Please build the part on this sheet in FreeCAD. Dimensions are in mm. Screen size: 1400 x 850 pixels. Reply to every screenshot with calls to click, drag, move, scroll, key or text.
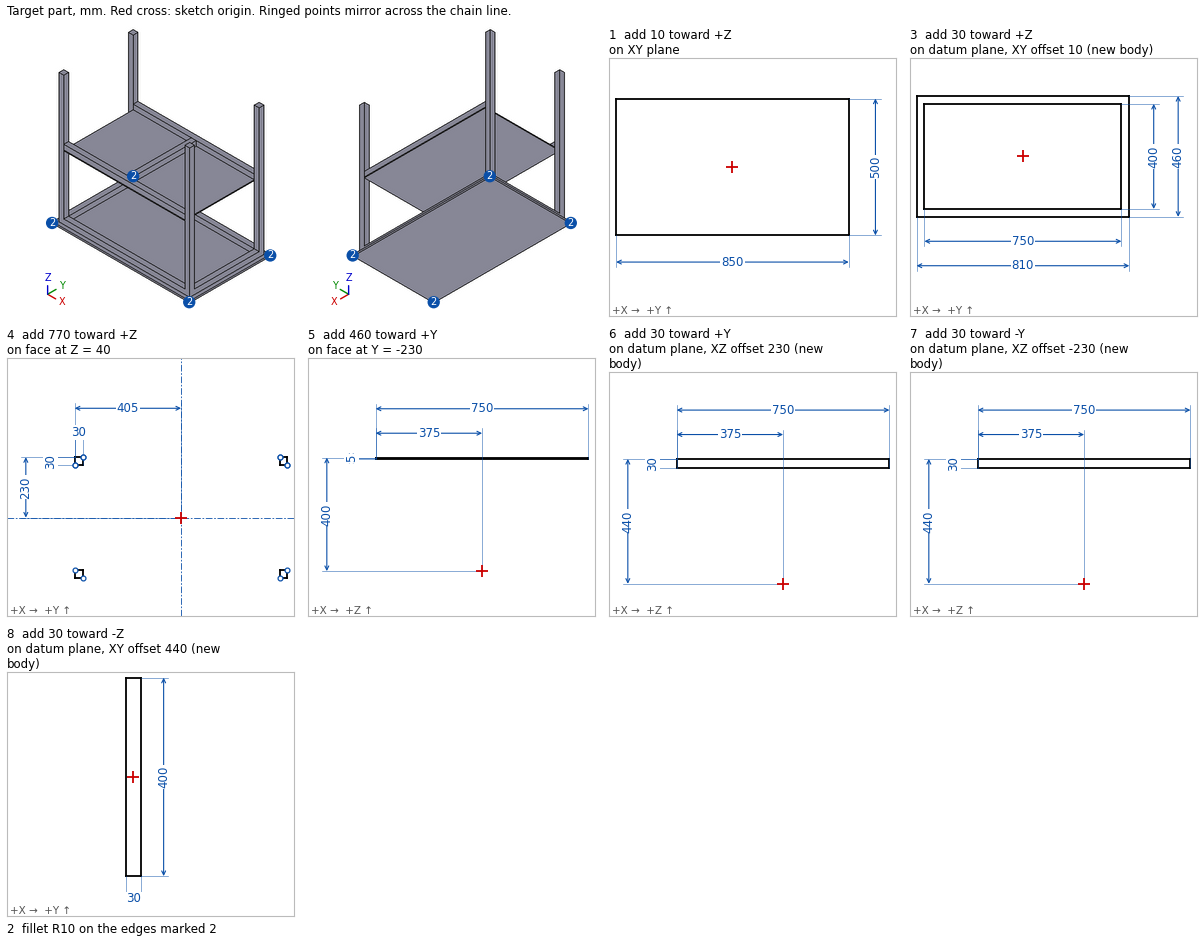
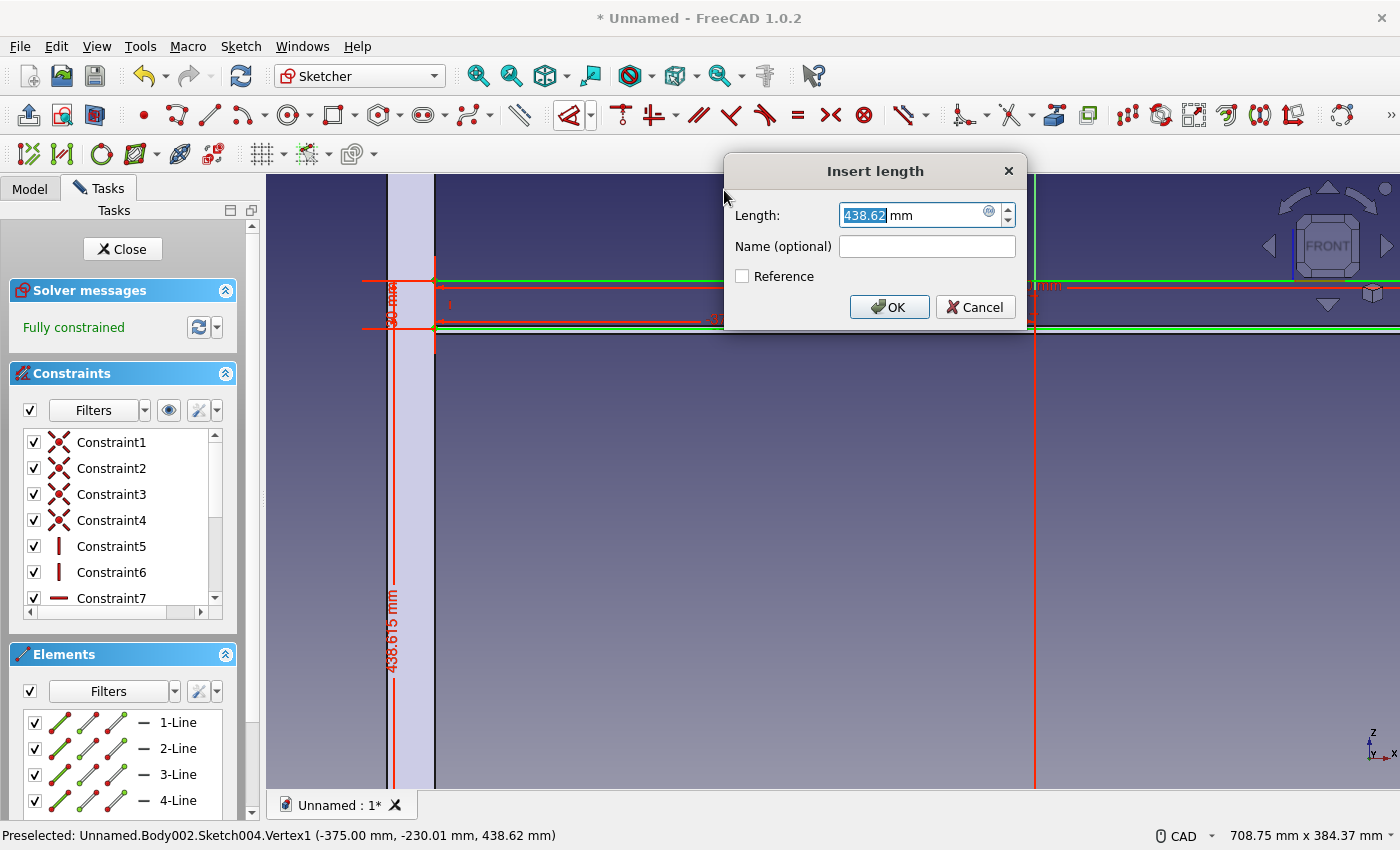
text(440)
key(Return)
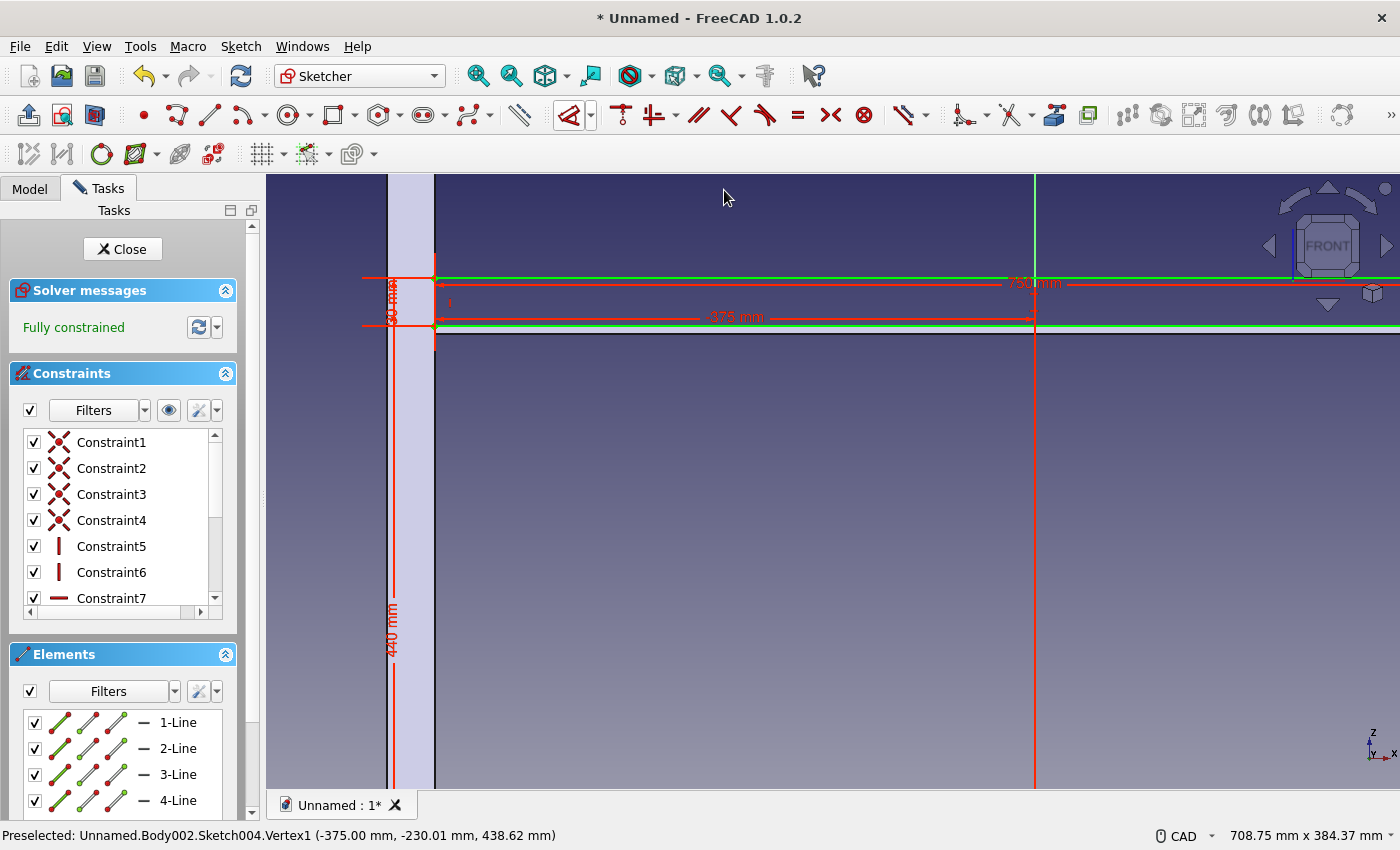
click(123, 249)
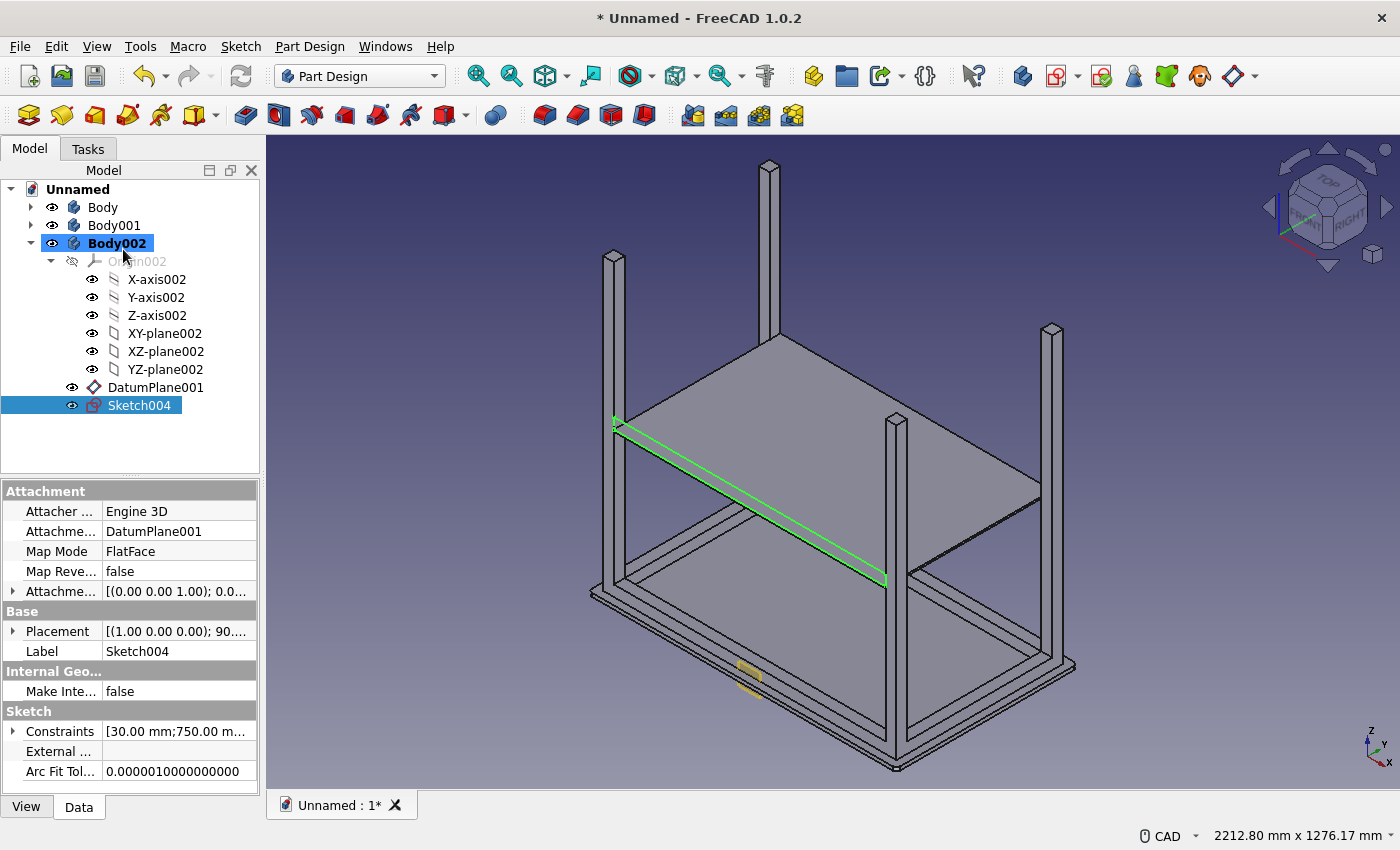
click(29, 116)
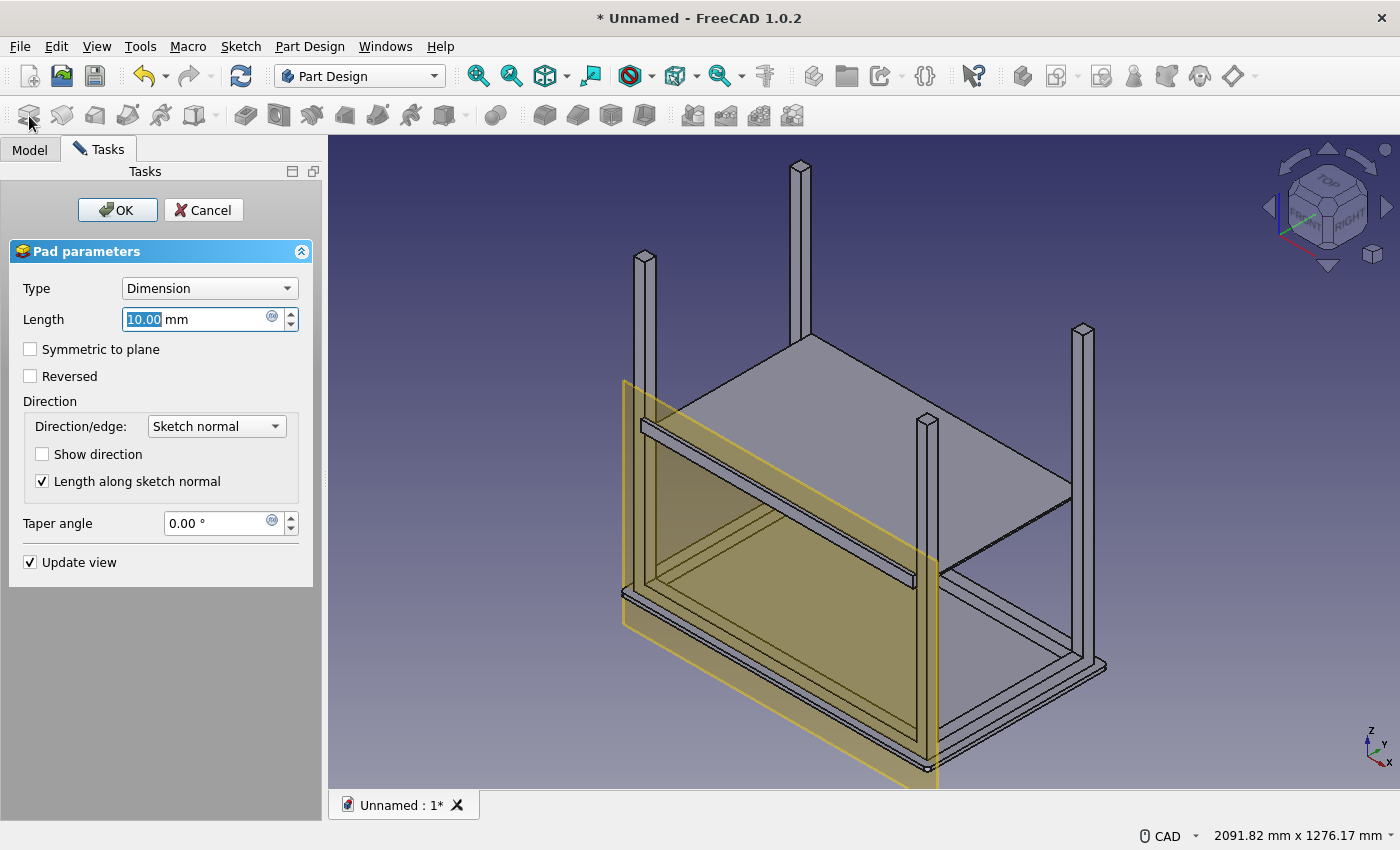
text(30)
key(Tab)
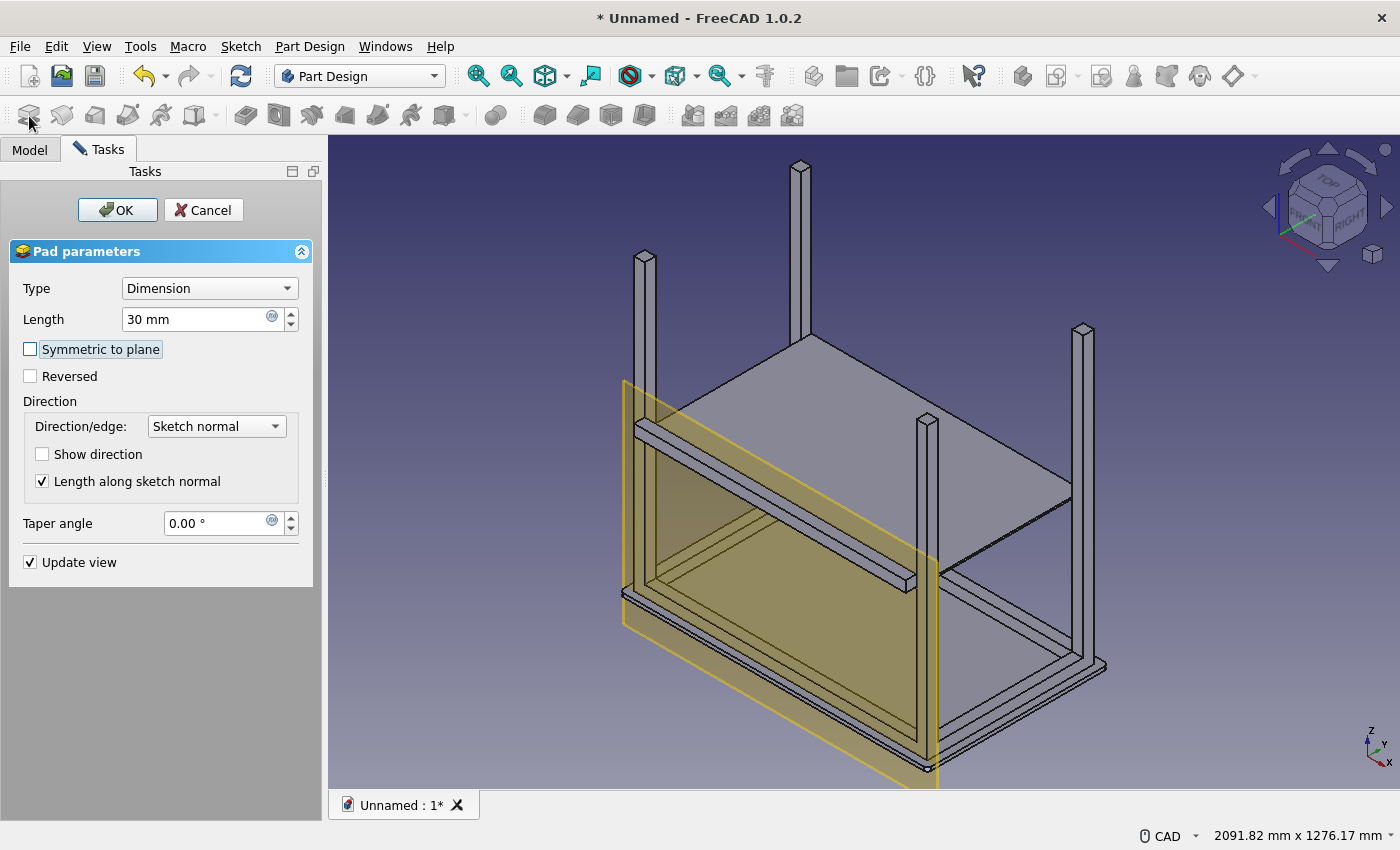
click(31, 376)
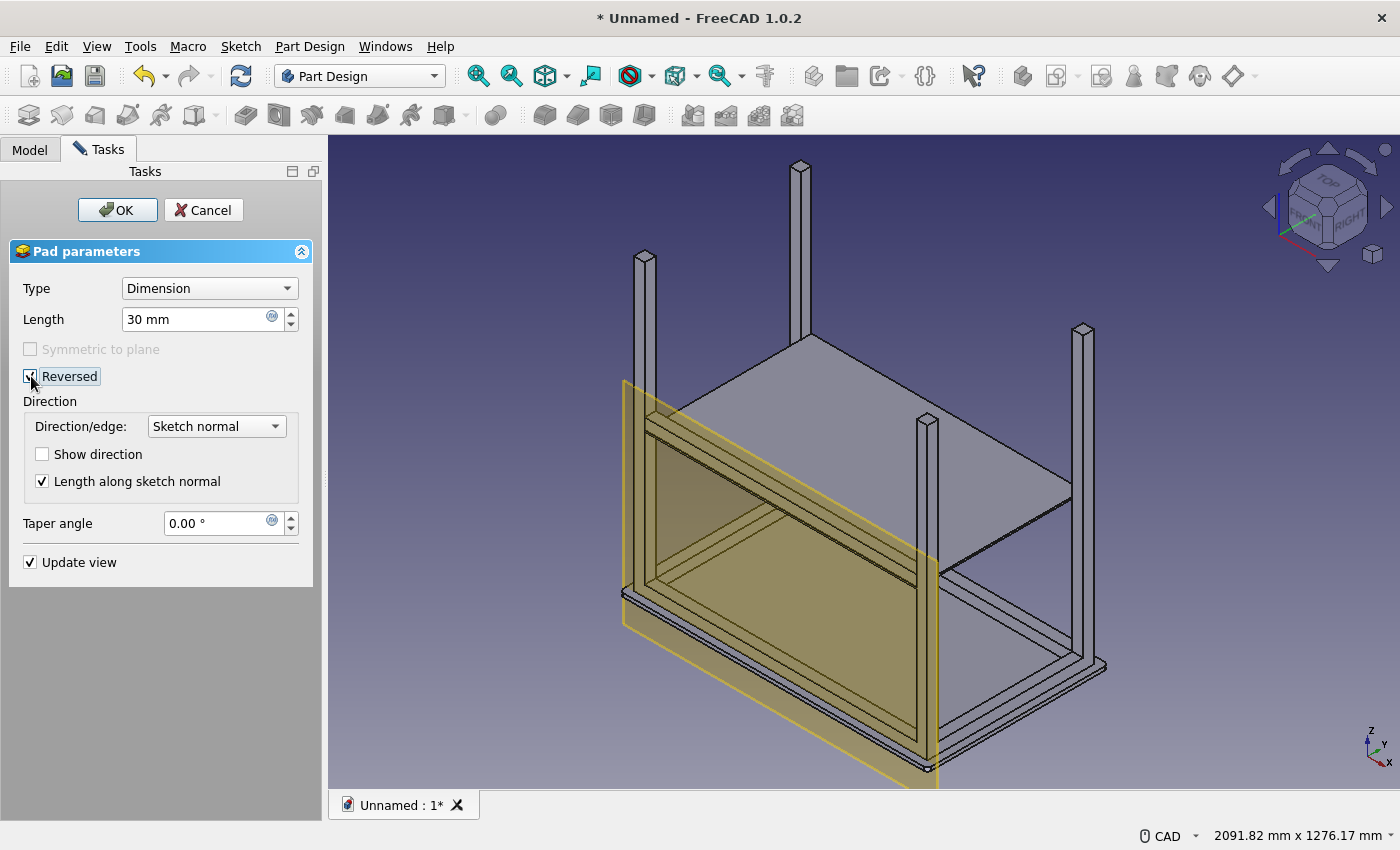
click(118, 210)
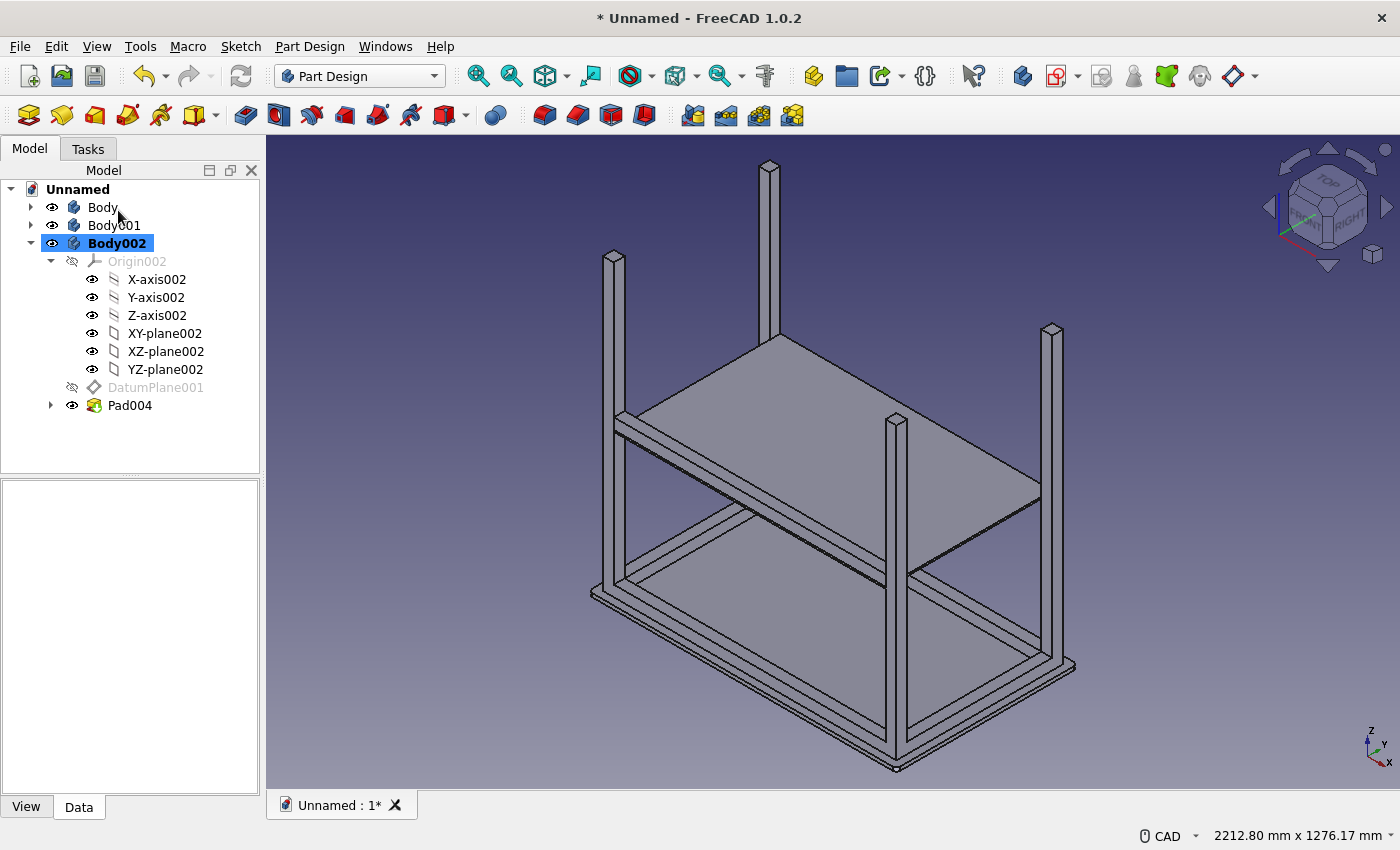
key(v)
key(f)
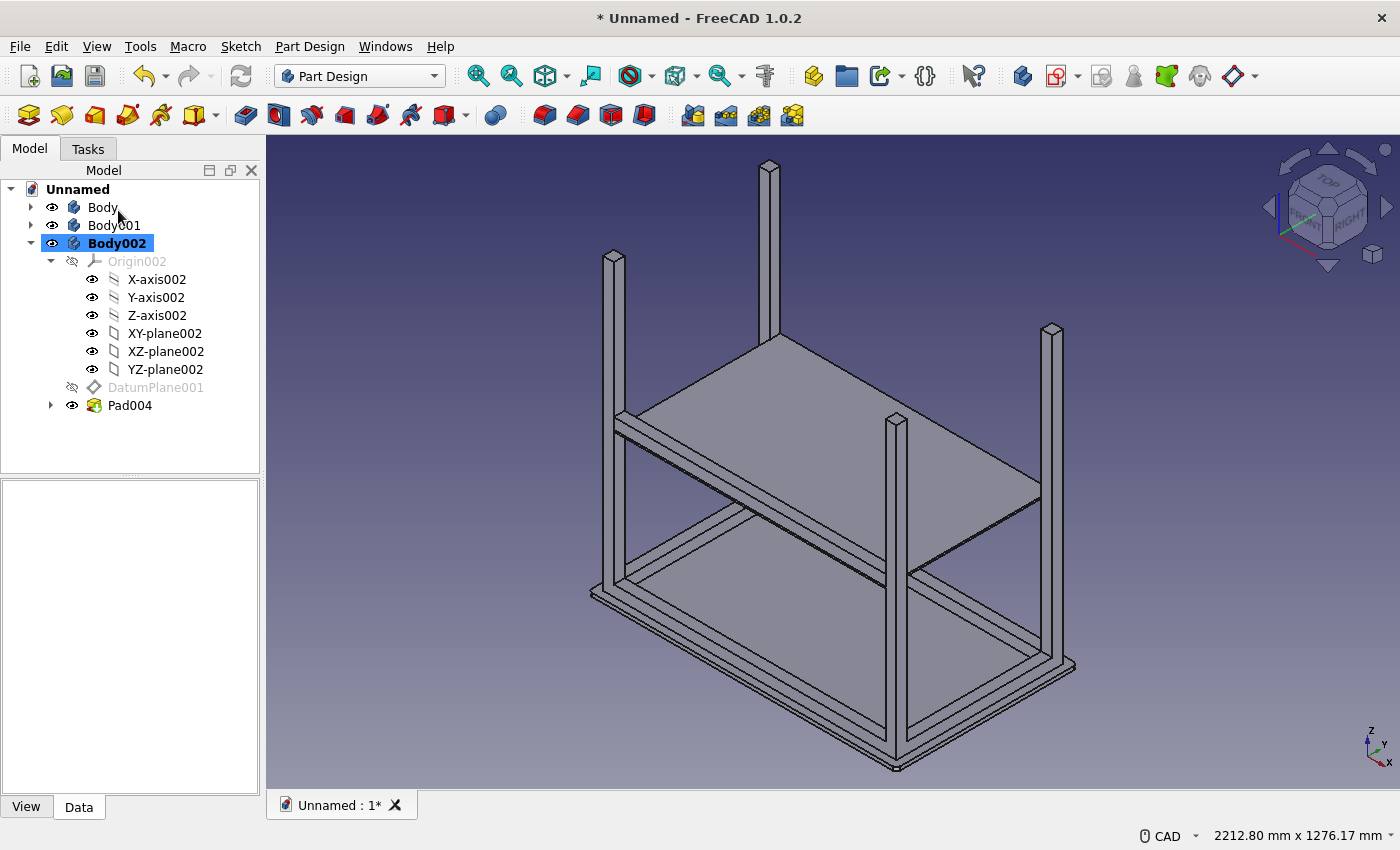
click(1023, 76)